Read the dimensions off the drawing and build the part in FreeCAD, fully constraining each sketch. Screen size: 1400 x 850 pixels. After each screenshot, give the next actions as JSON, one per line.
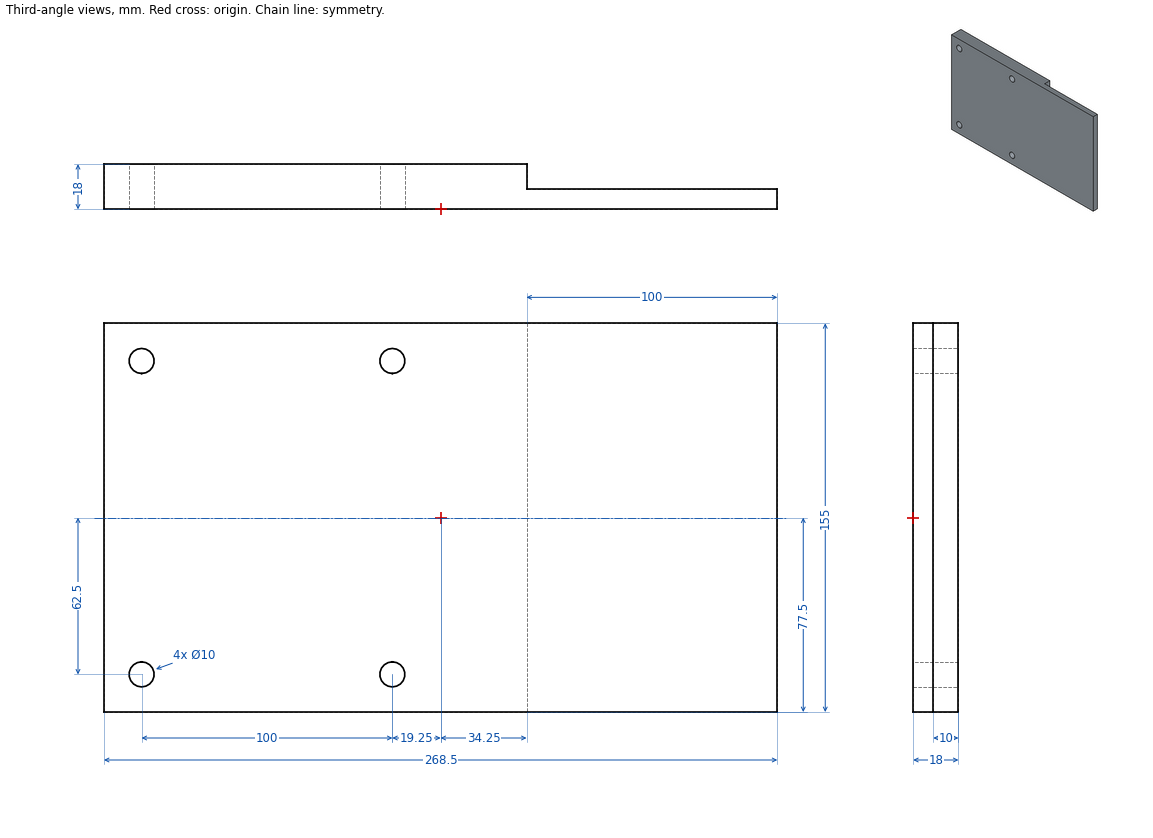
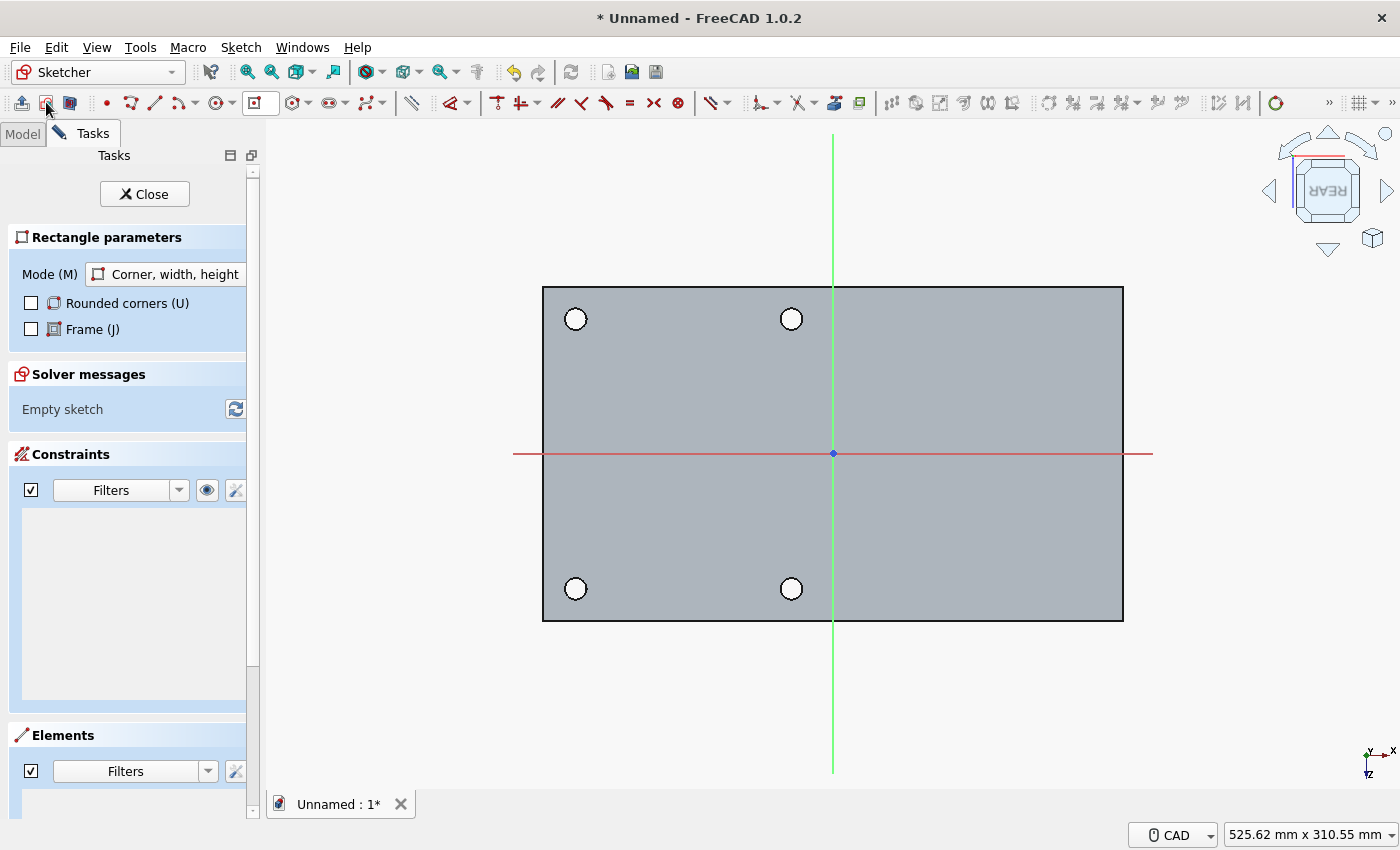
{"action": "left_click", "coordinate": [907, 287]}
{"action": "left_click", "coordinate": [1123, 621]}
{"action": "key", "text": "Escape"}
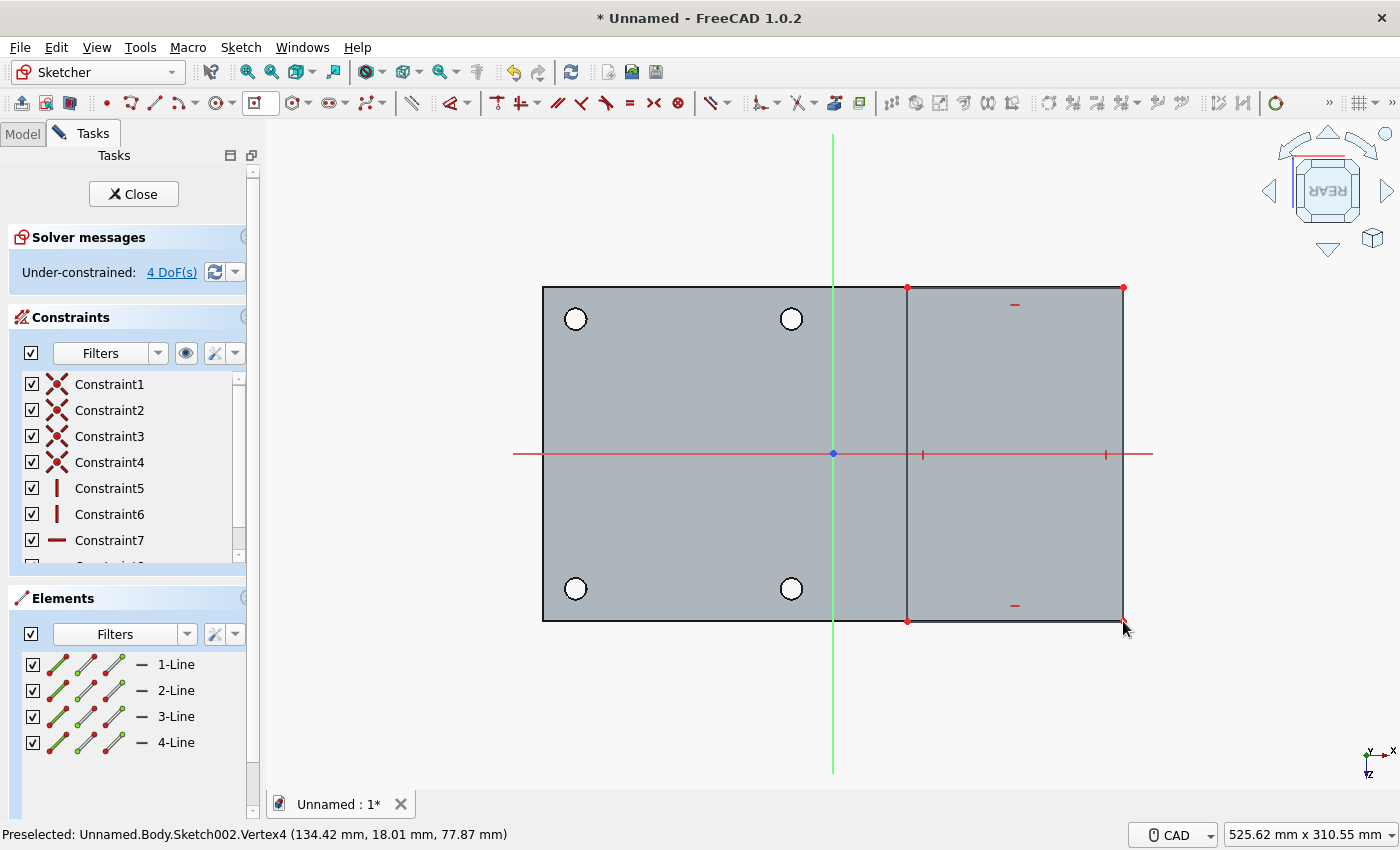
{"action": "left_click", "coordinate": [450, 104]}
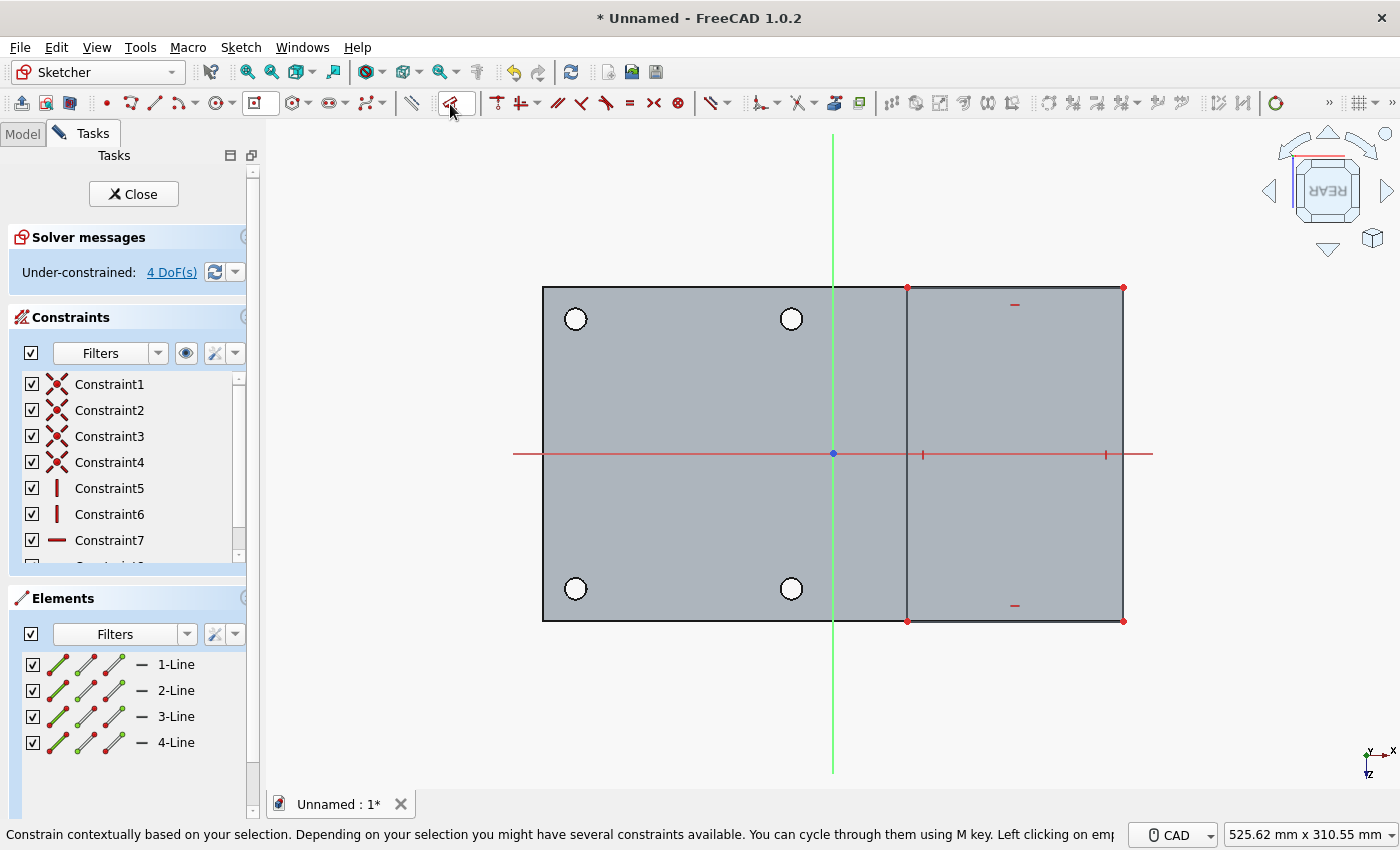
{"action": "left_click", "coordinate": [907, 388]}
{"action": "left_click", "coordinate": [873, 378]}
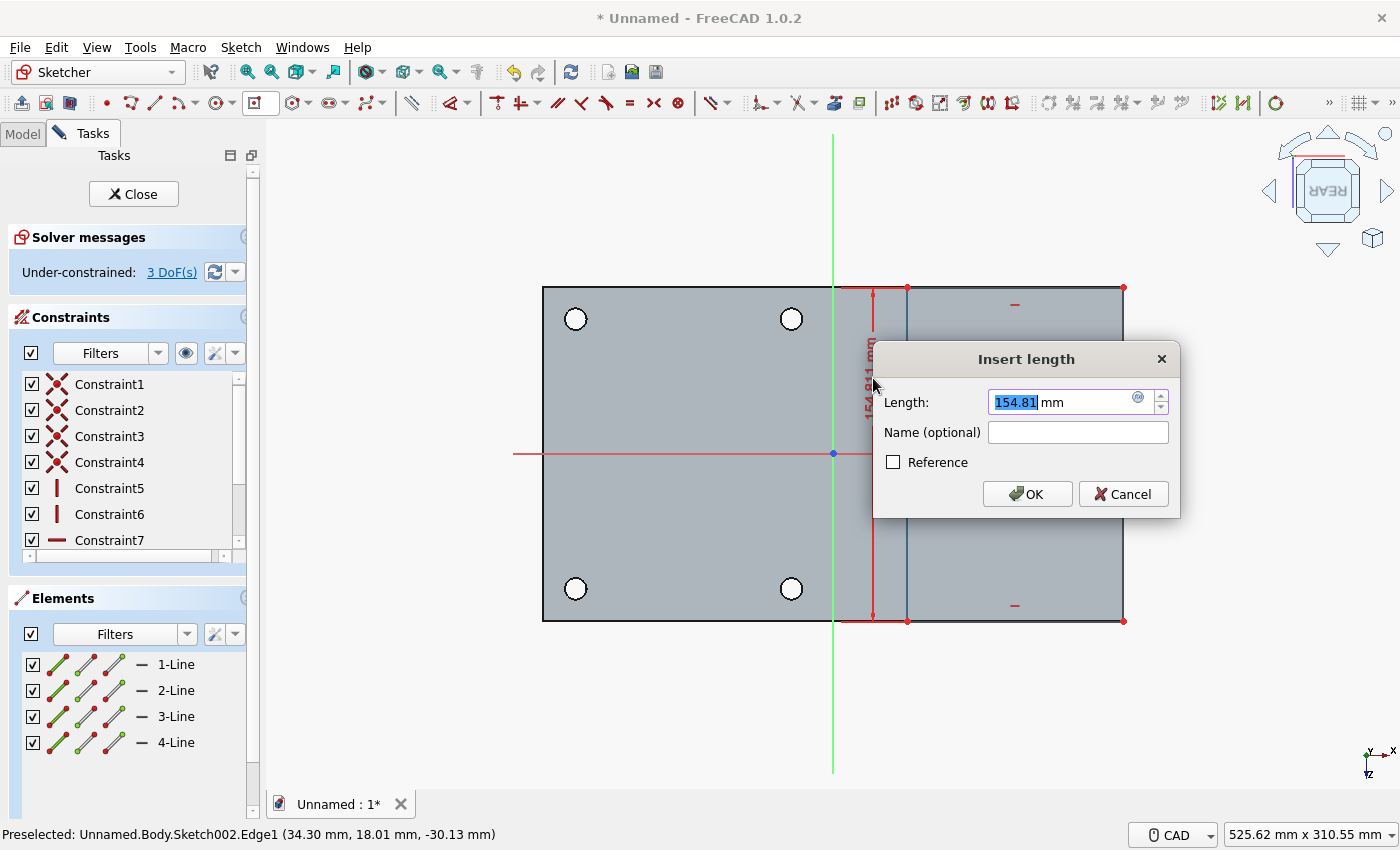
{"action": "type", "text": "155"}
{"action": "key", "text": "Return"}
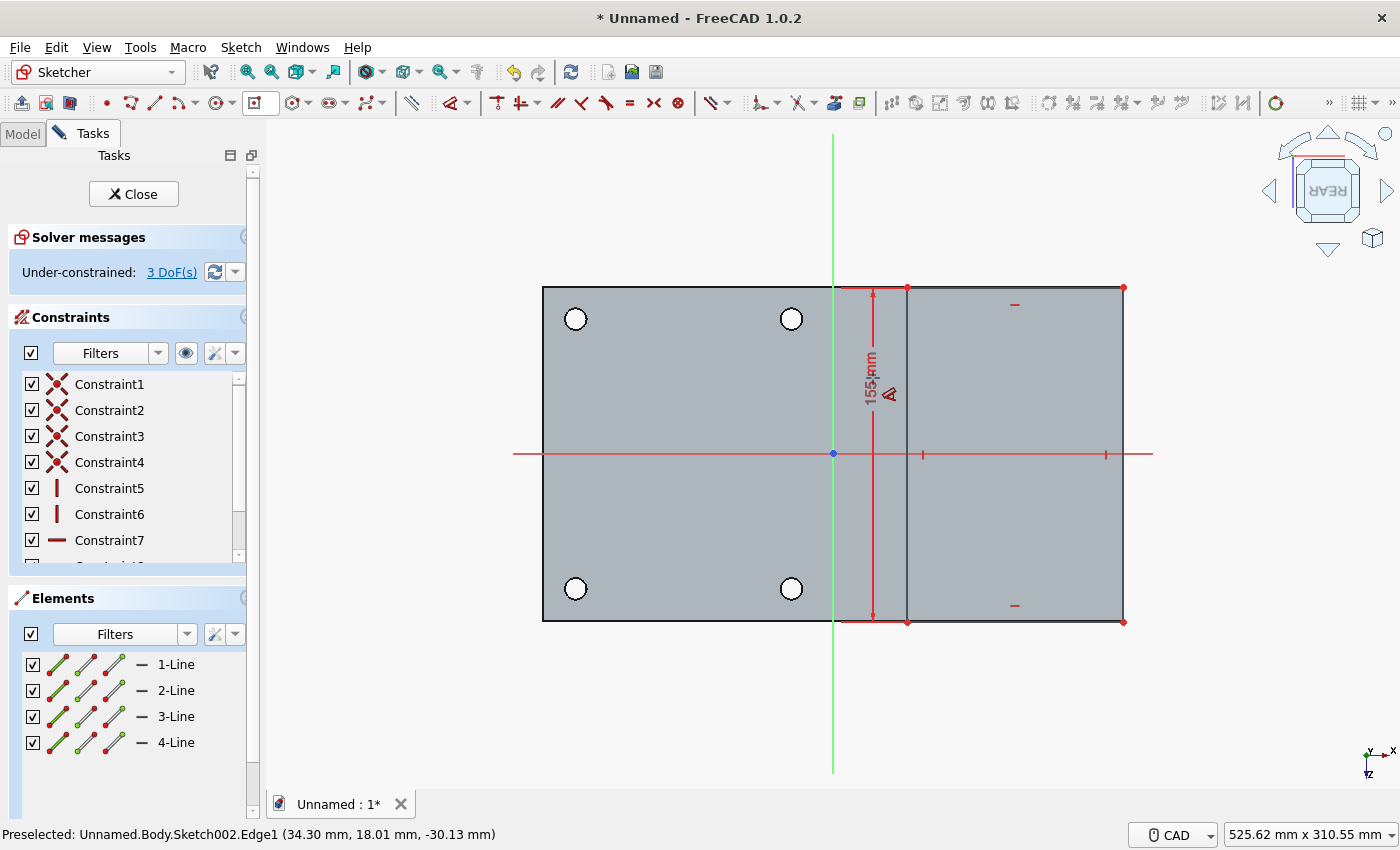
{"action": "left_click", "coordinate": [972, 622]}
{"action": "left_click", "coordinate": [1015, 656]}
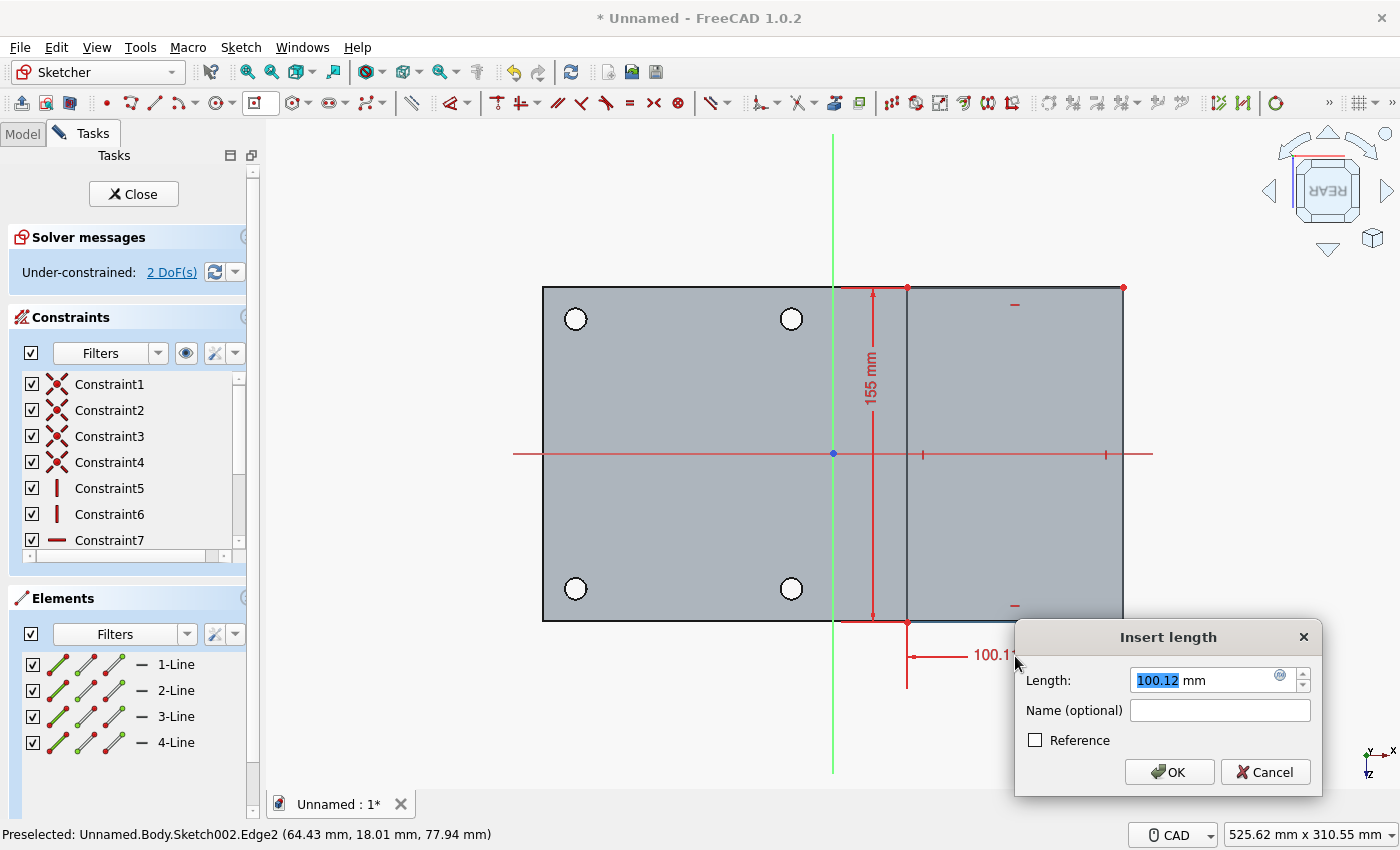
{"action": "type", "text": "100"}
{"action": "key", "text": "Return"}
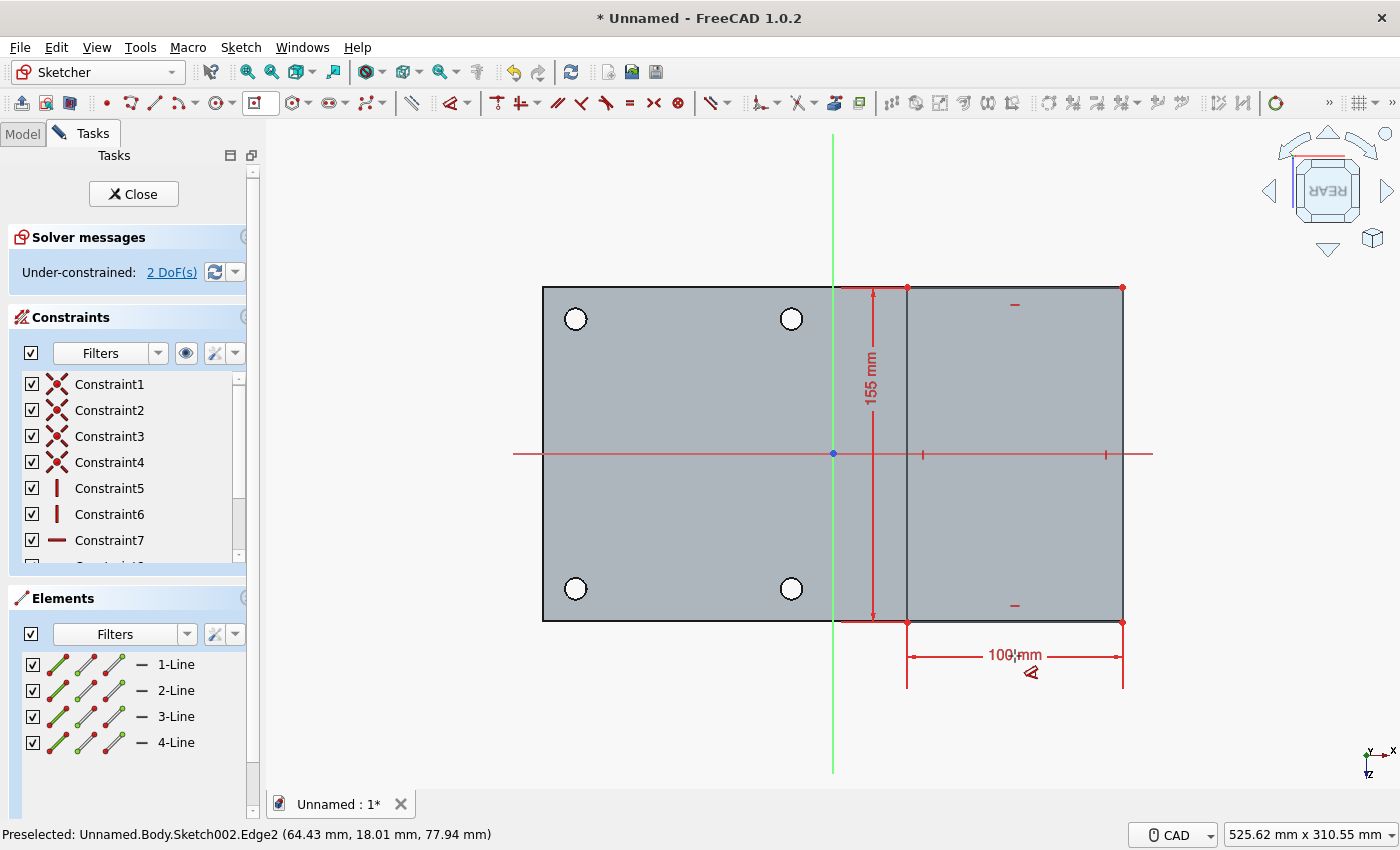
{"action": "left_click", "coordinate": [907, 288]}
{"action": "left_click", "coordinate": [799, 371]}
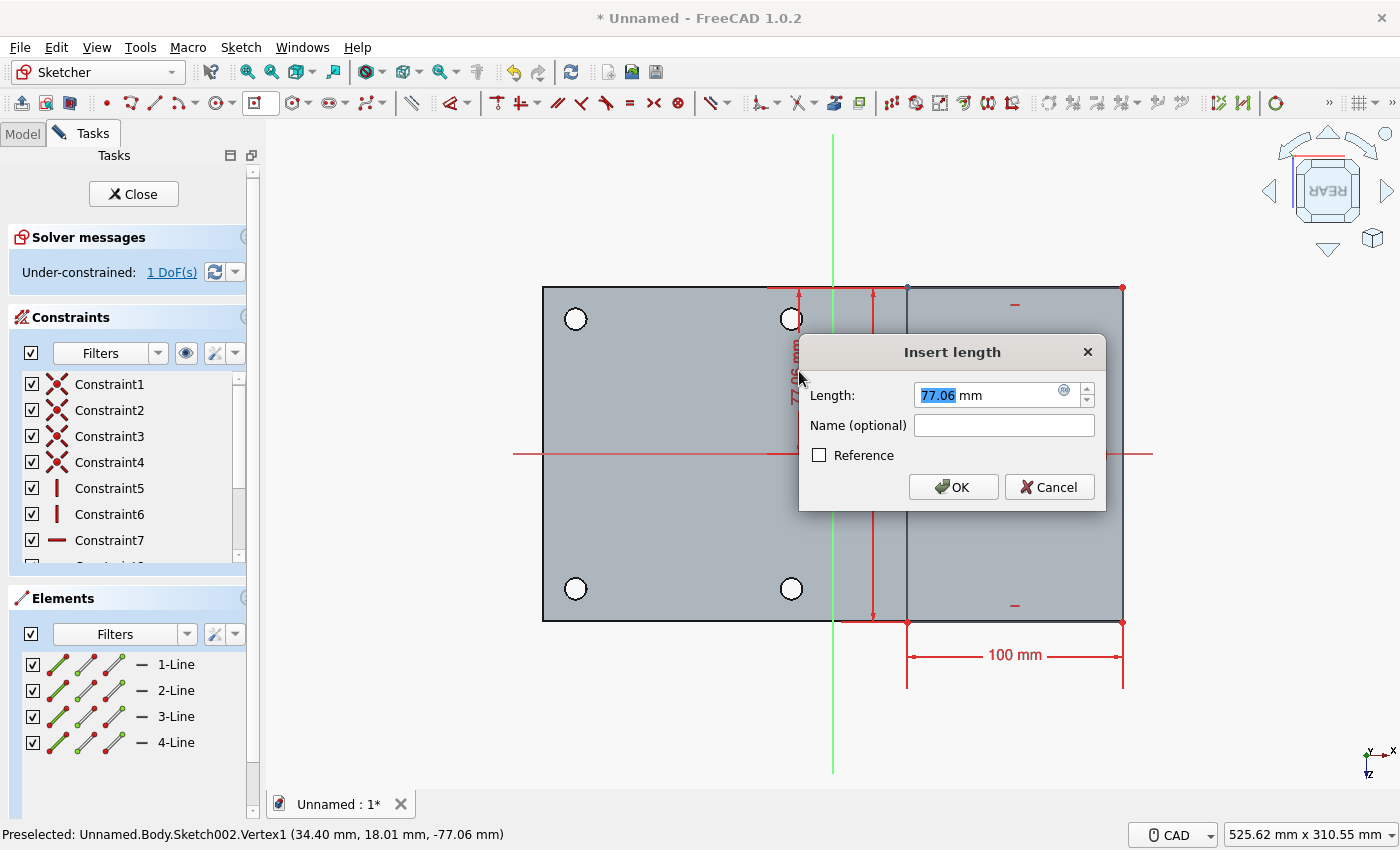
{"action": "type", "text": "77.5"}
{"action": "key", "text": "Return"}